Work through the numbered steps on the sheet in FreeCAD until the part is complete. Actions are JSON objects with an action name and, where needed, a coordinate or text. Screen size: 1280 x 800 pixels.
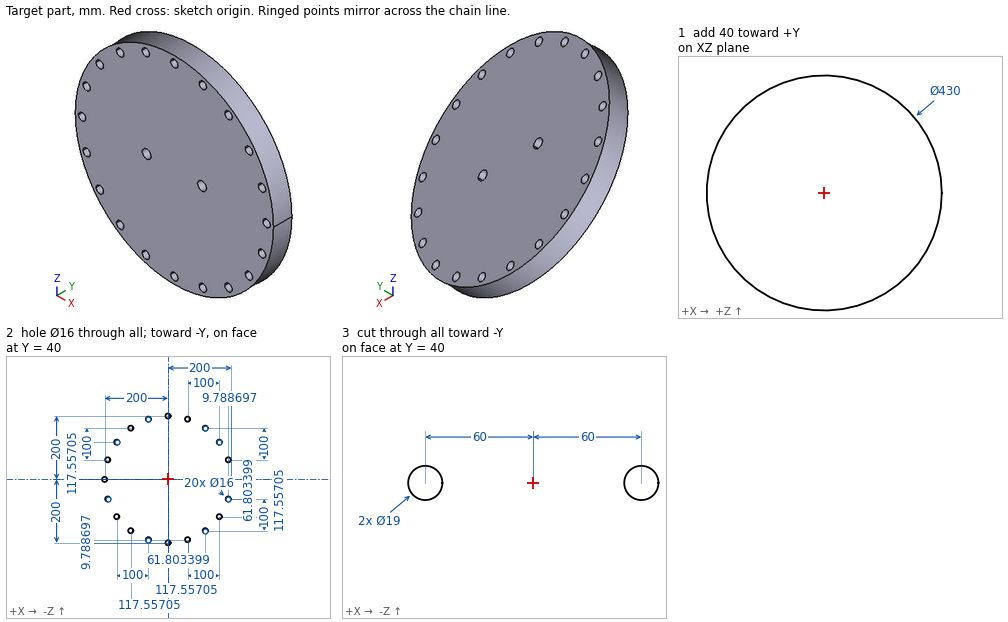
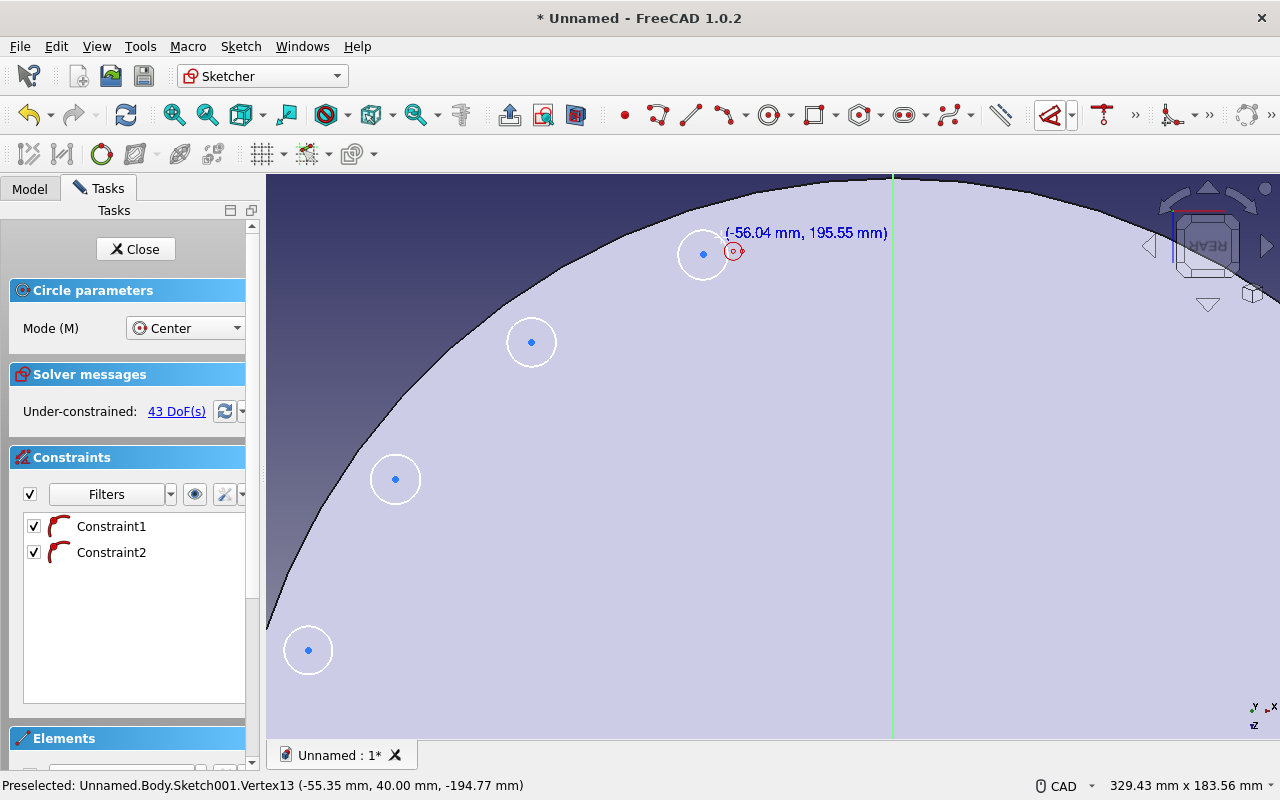
{"action": "left_click", "coordinate": [893, 224]}
{"action": "left_click", "coordinate": [911, 207]}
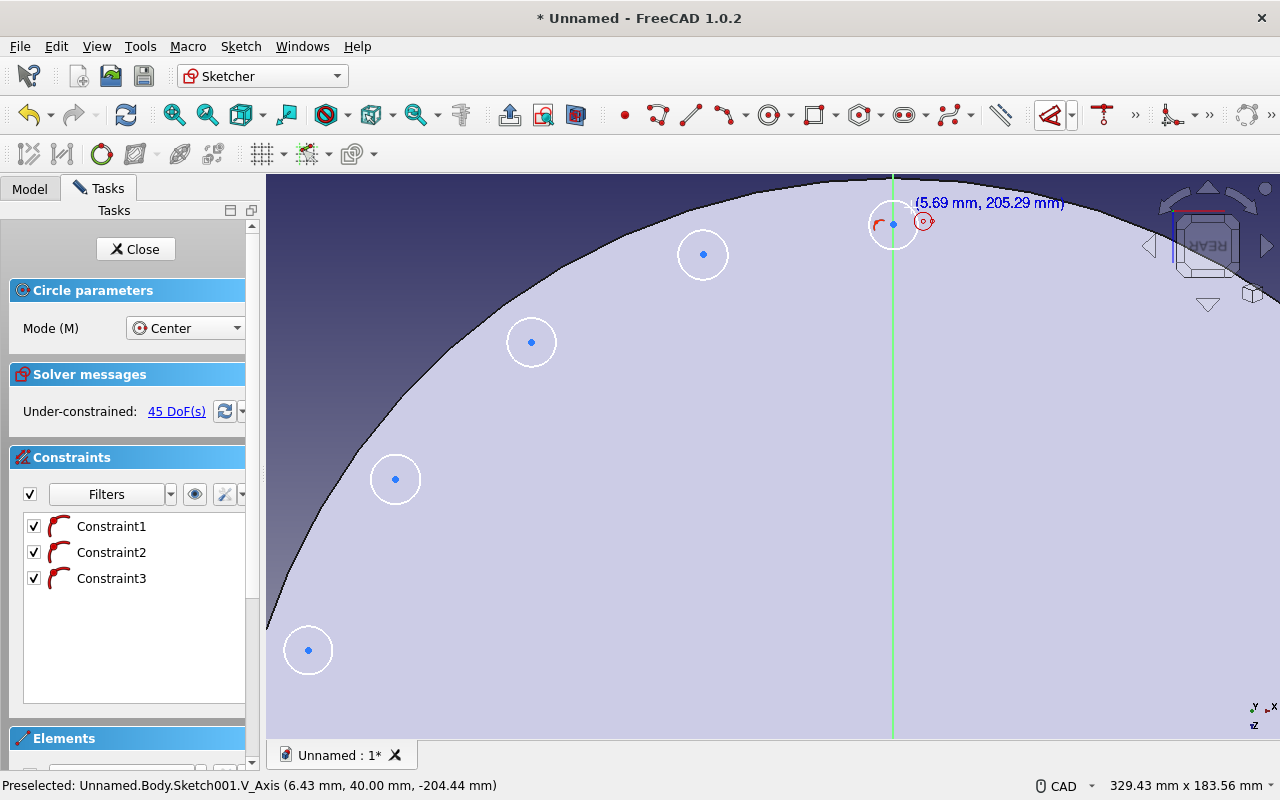
{"action": "left_click", "coordinate": [1084, 254]}
{"action": "left_click", "coordinate": [1101, 237]}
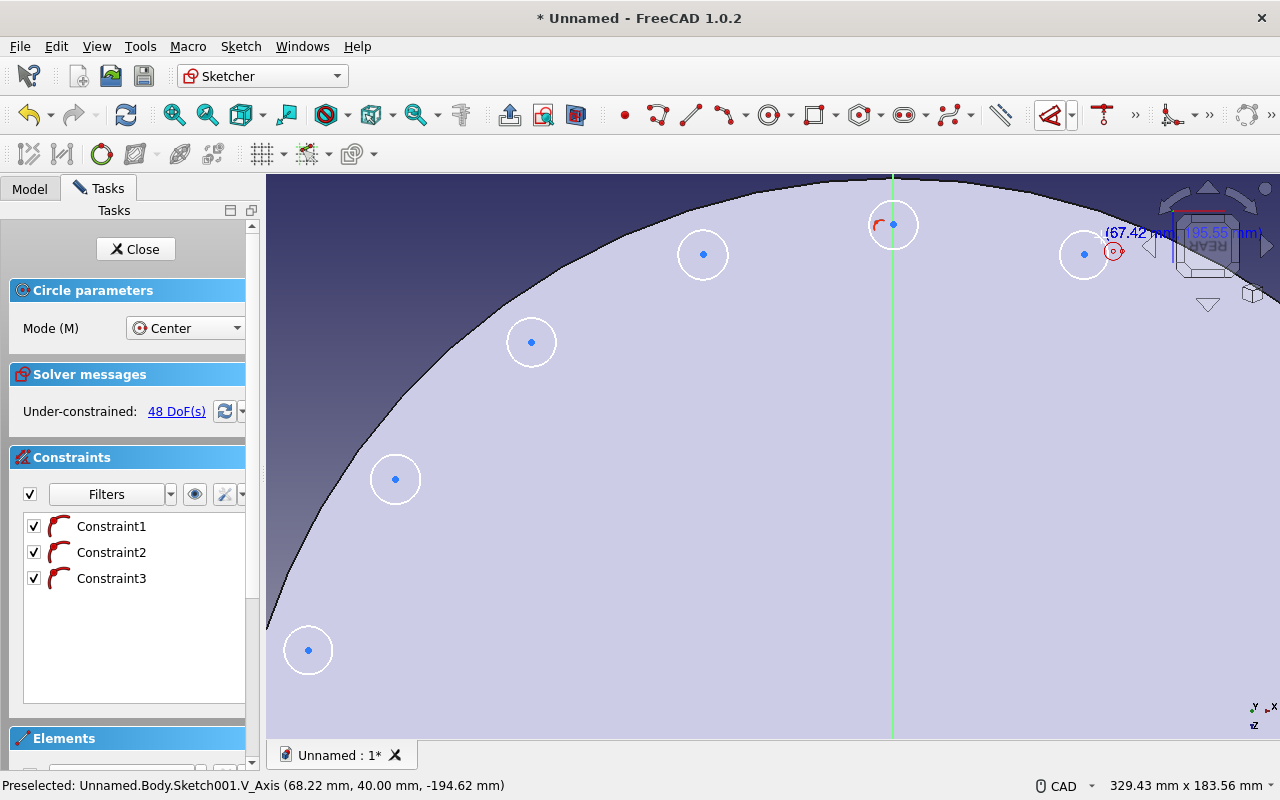
{"action": "scroll", "coordinate": [623, 291], "scroll_direction": "down", "scroll_amount": 6}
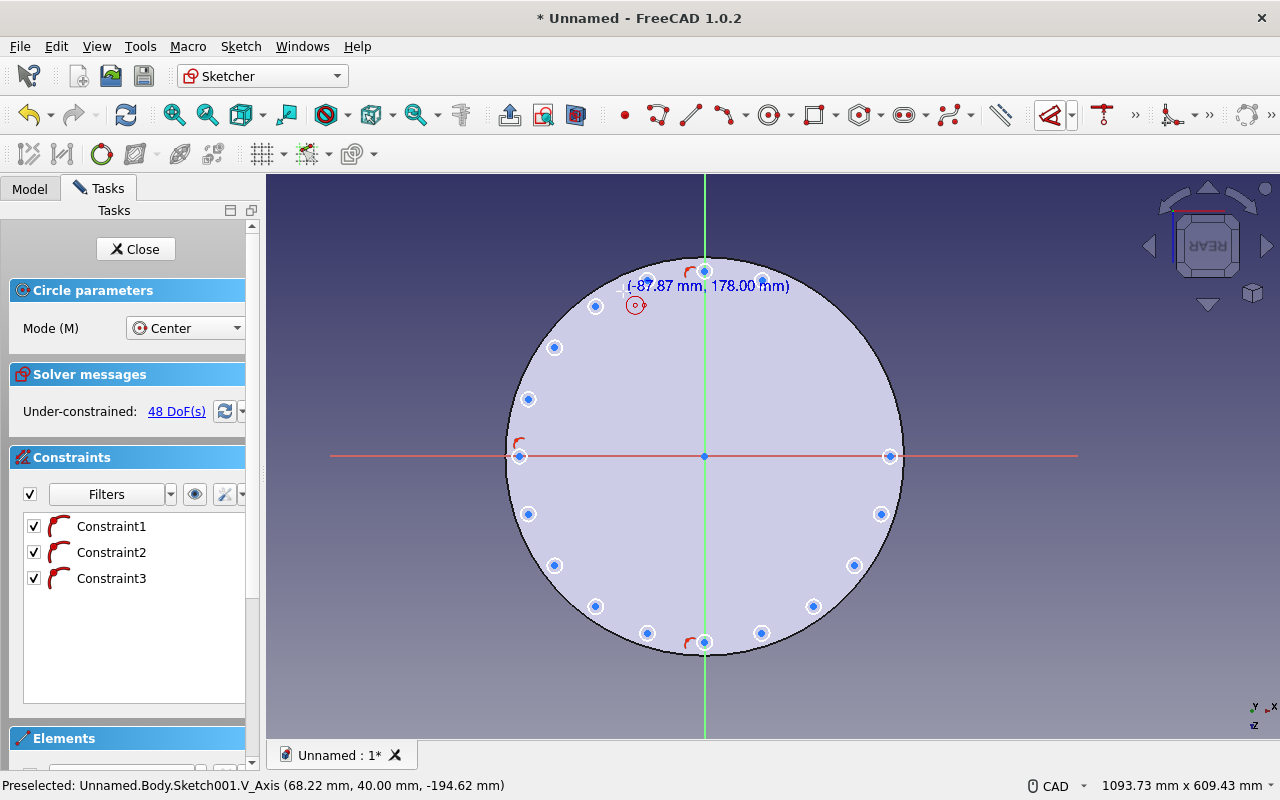
{"action": "scroll", "coordinate": [814, 306], "scroll_direction": "up", "scroll_amount": 6}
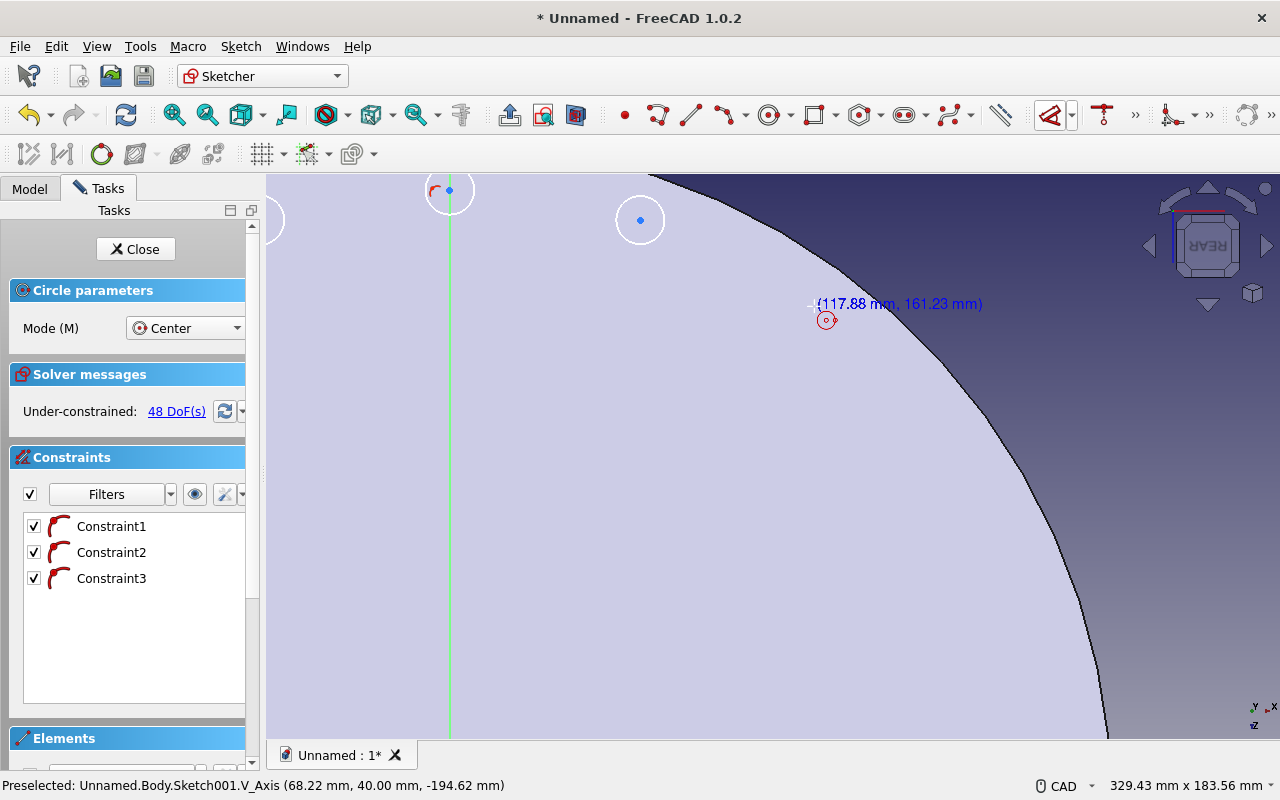
{"action": "left_click", "coordinate": [812, 307]}
{"action": "left_click", "coordinate": [829, 290]}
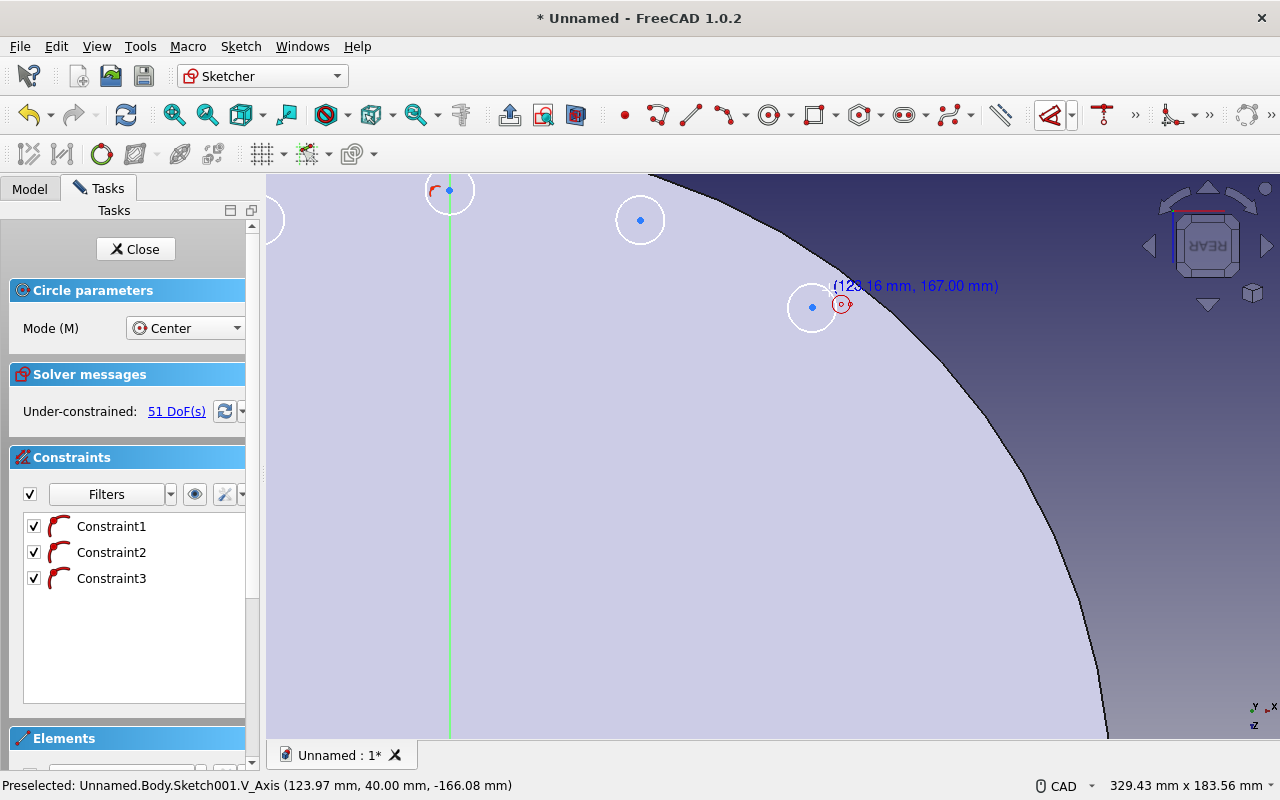
{"action": "left_click", "coordinate": [948, 443]}
{"action": "left_click", "coordinate": [965, 426]}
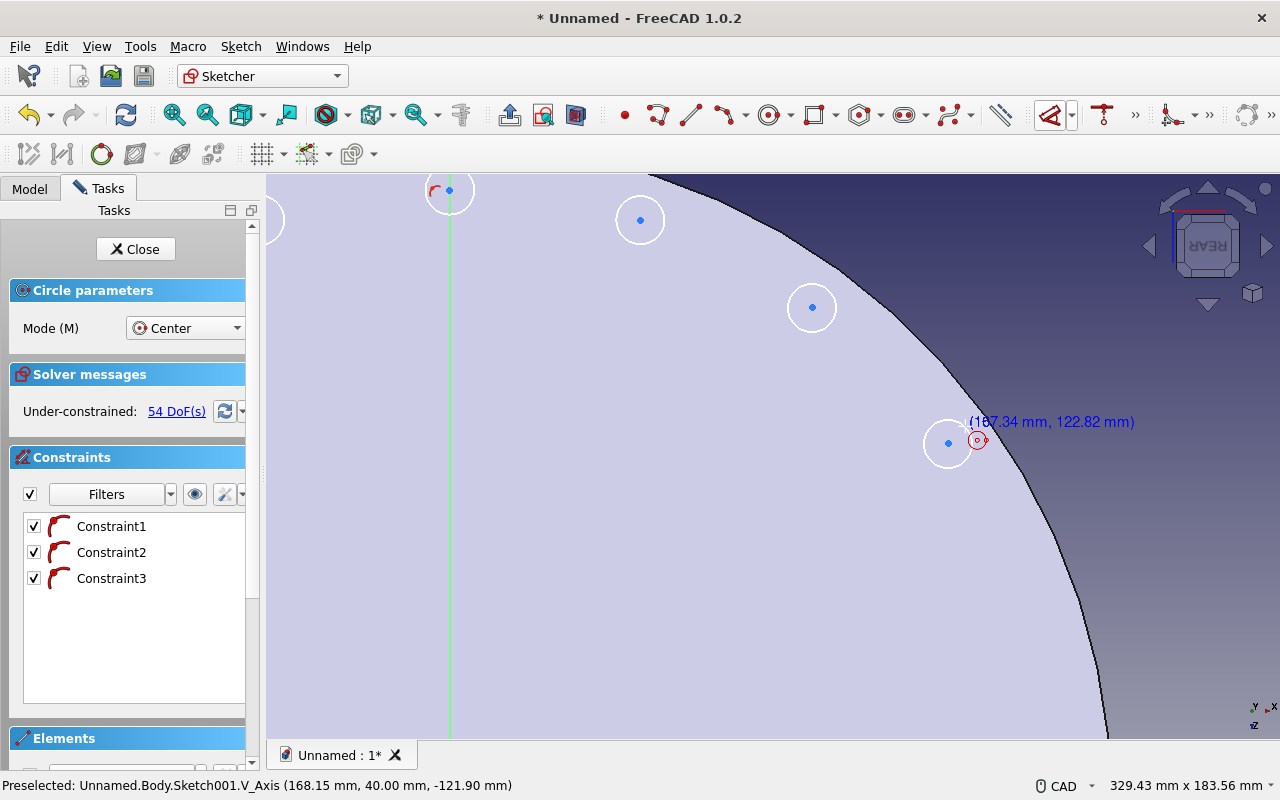
{"action": "left_click", "coordinate": [1035, 615]}
{"action": "left_click", "coordinate": [1053, 597]}
{"action": "key", "text": "Escape"}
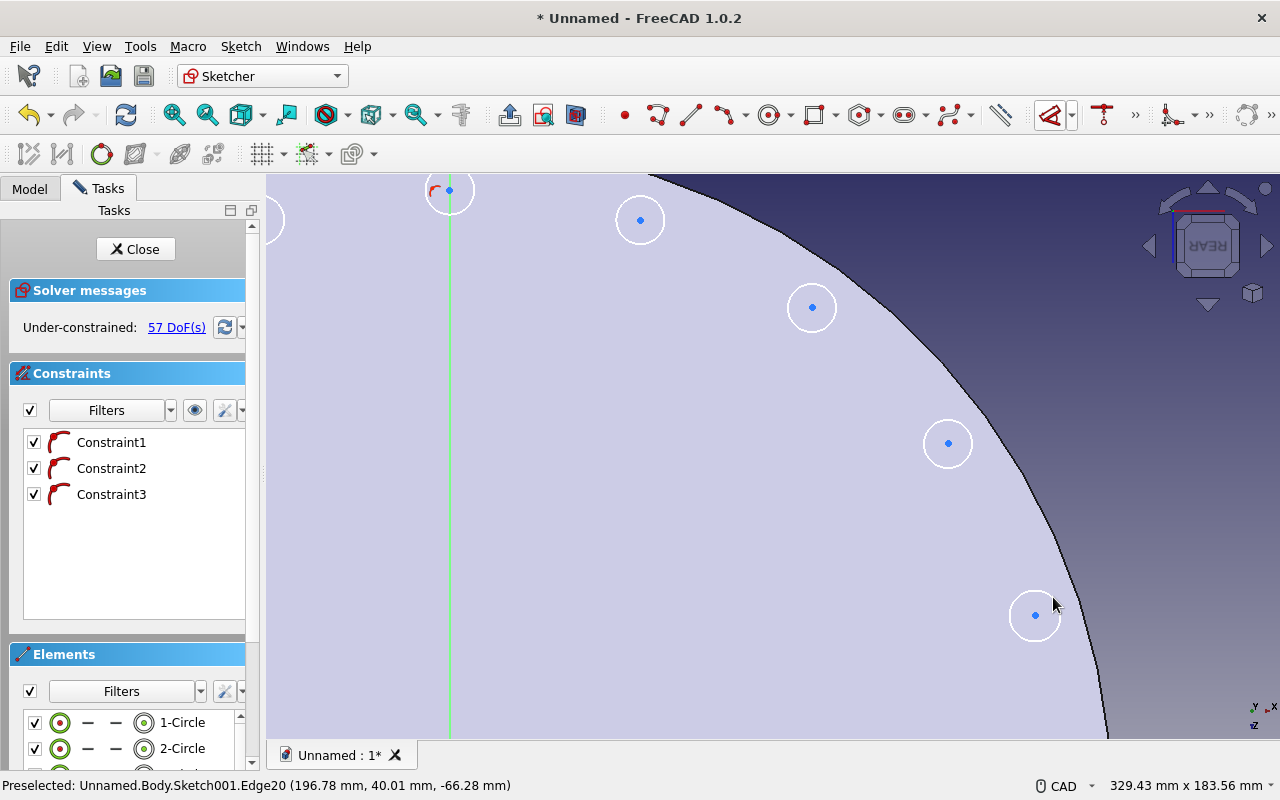
{"action": "scroll", "coordinate": [814, 306], "scroll_direction": "down", "scroll_amount": 6}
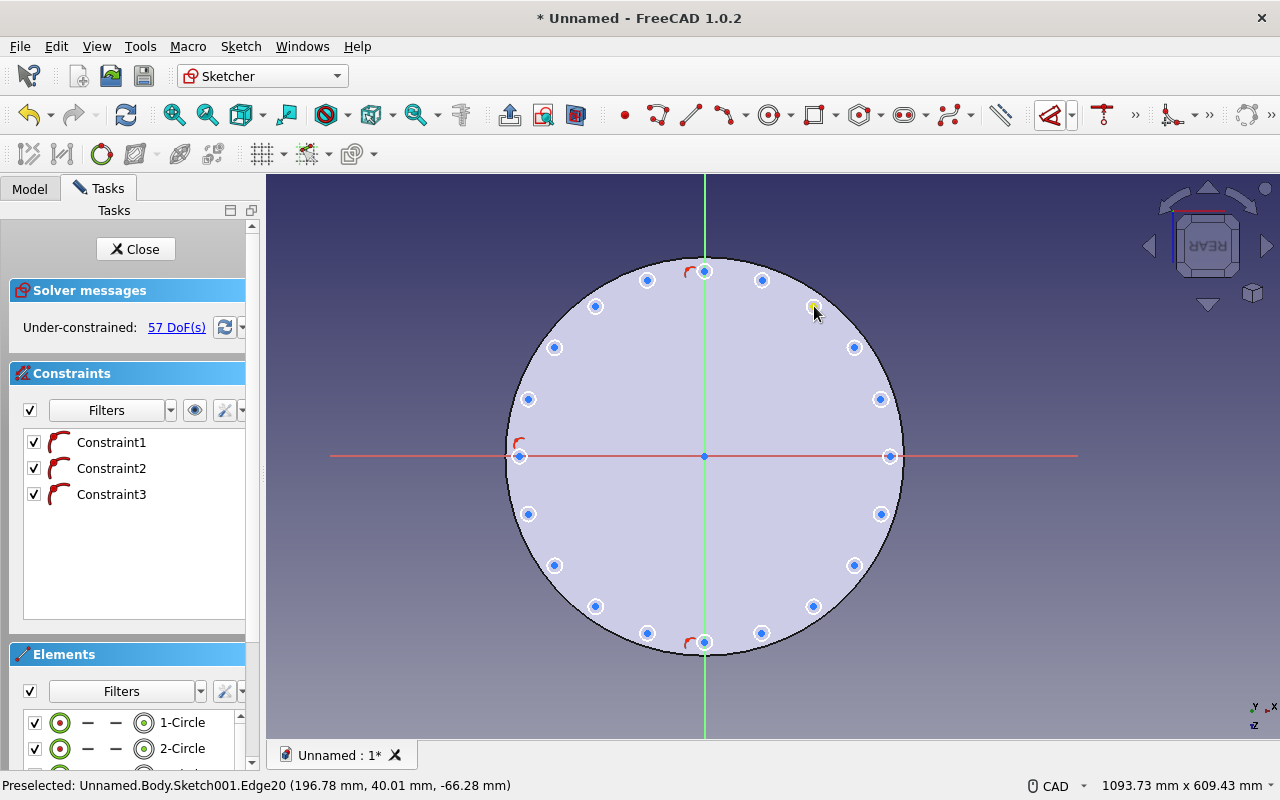
{"action": "scroll", "coordinate": [895, 451], "scroll_direction": "up", "scroll_amount": 6}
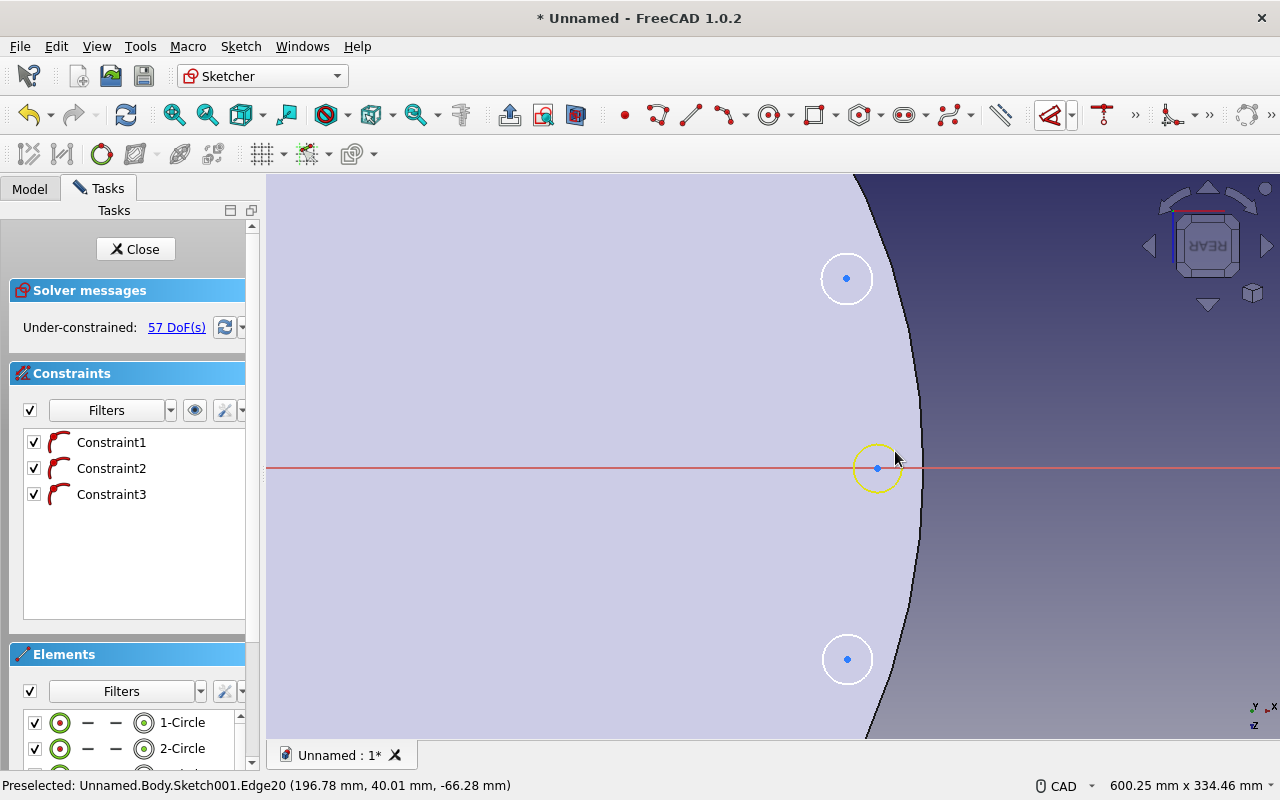
{"action": "left_click", "coordinate": [895, 451]}